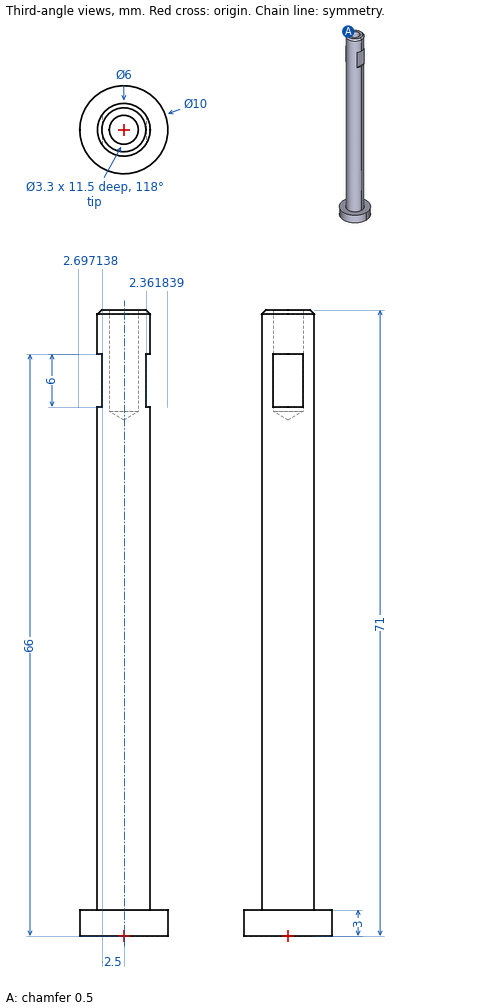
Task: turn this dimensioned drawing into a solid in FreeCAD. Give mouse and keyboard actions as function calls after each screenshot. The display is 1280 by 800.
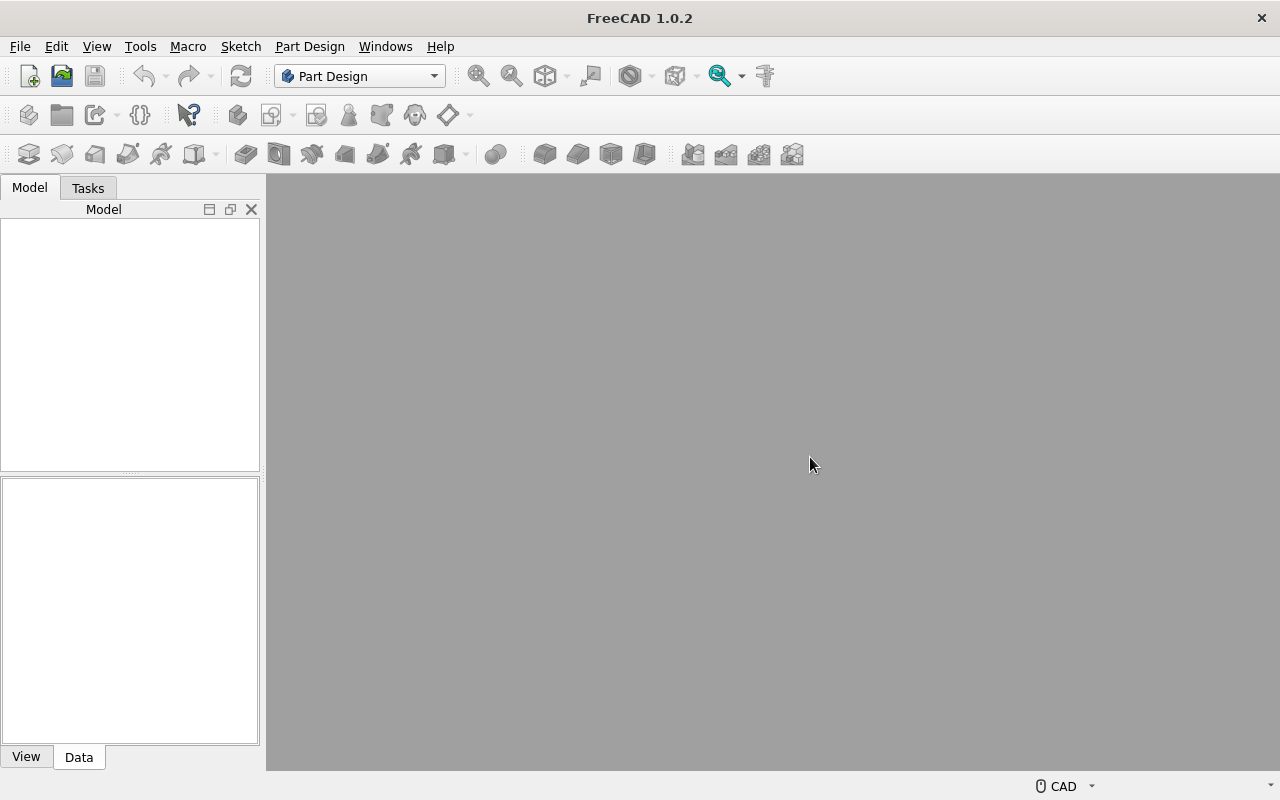
key(ctrl+n)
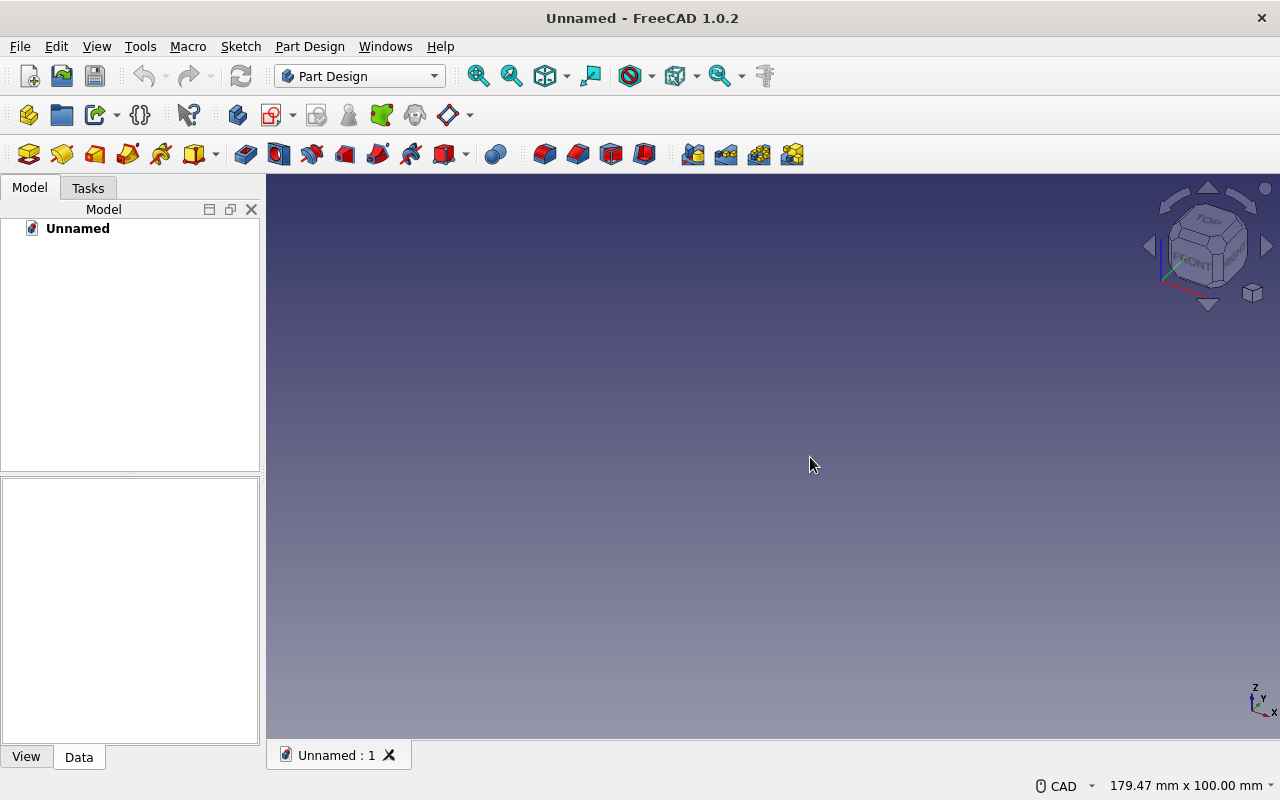
click(270, 116)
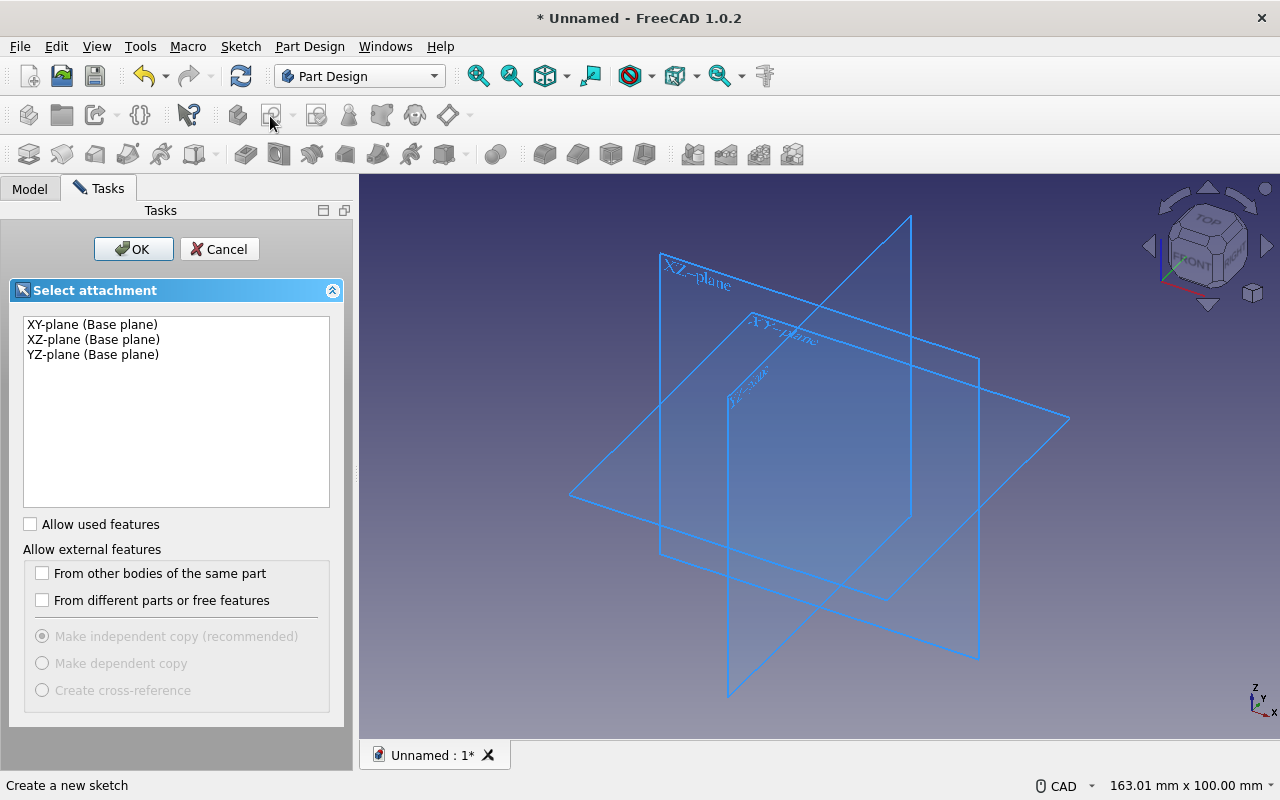
click(84, 324)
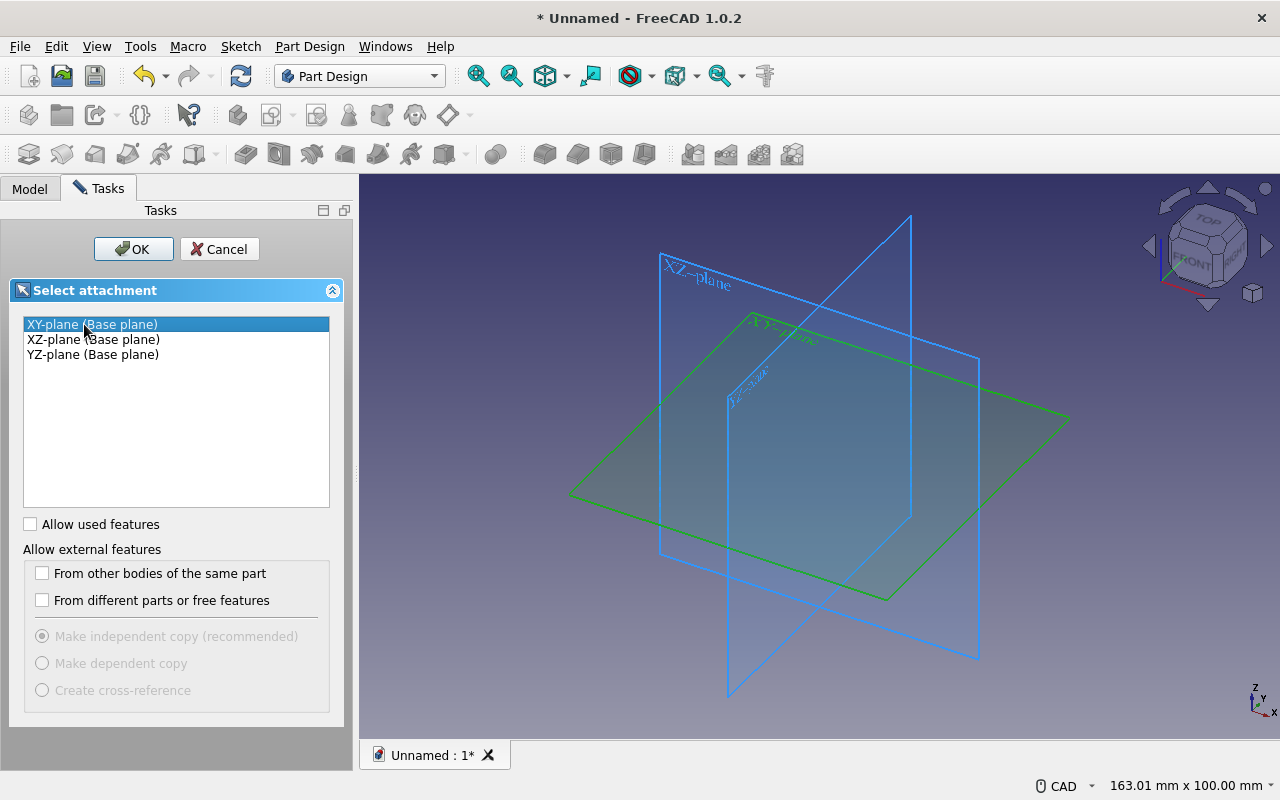
click(134, 249)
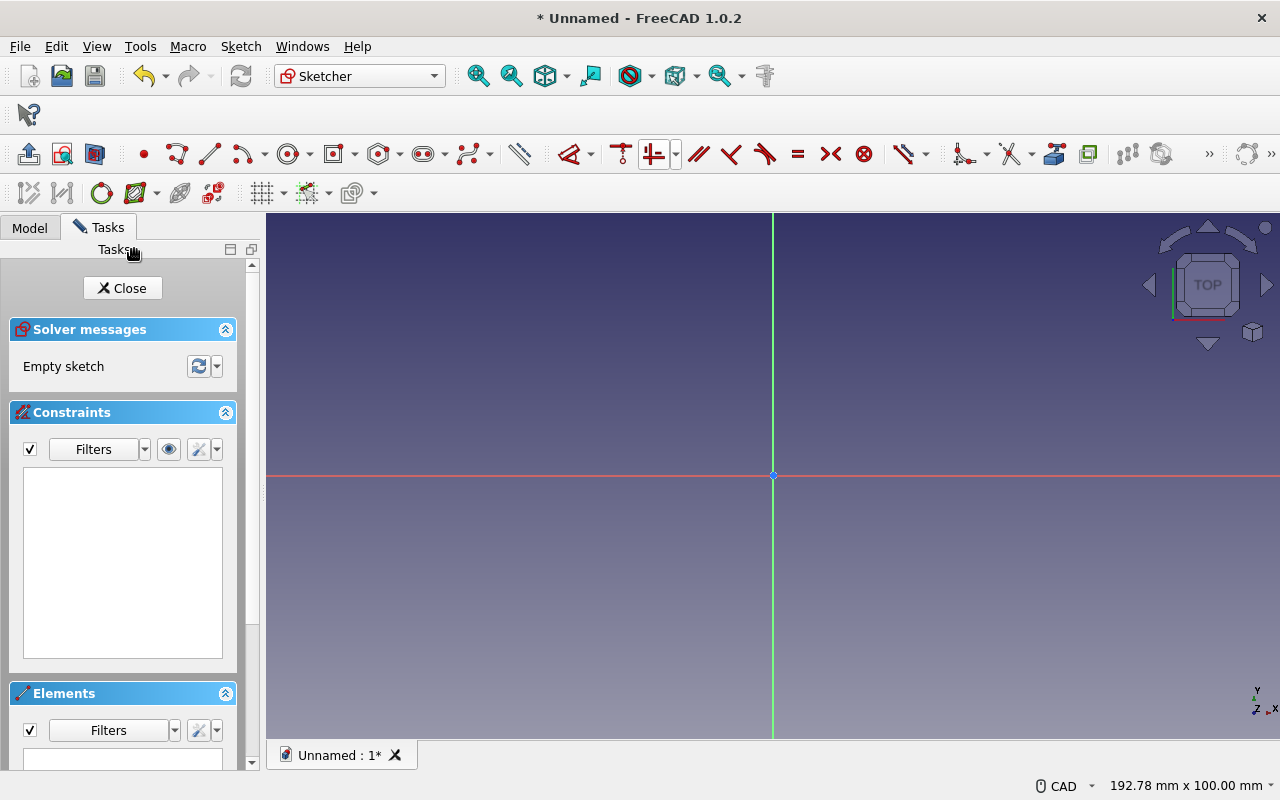
scroll(780, 476, up, 12)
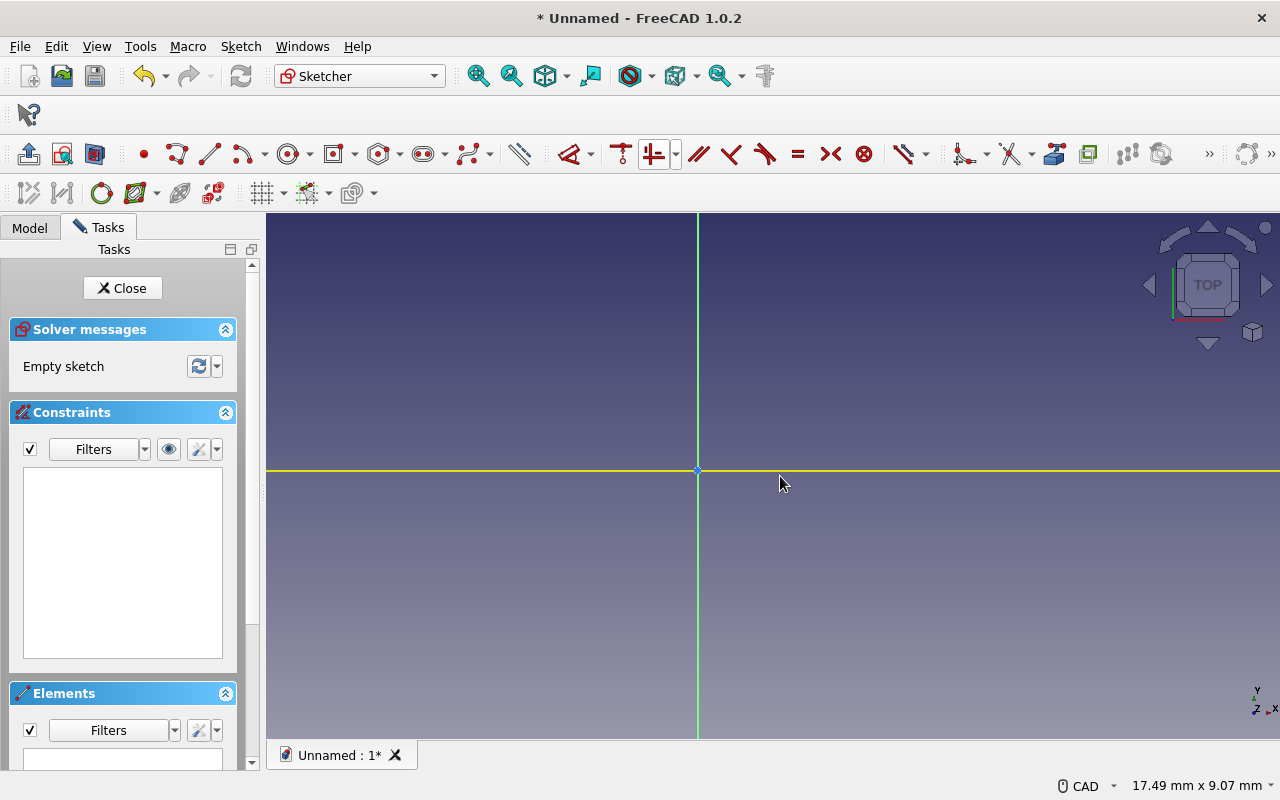
click(288, 154)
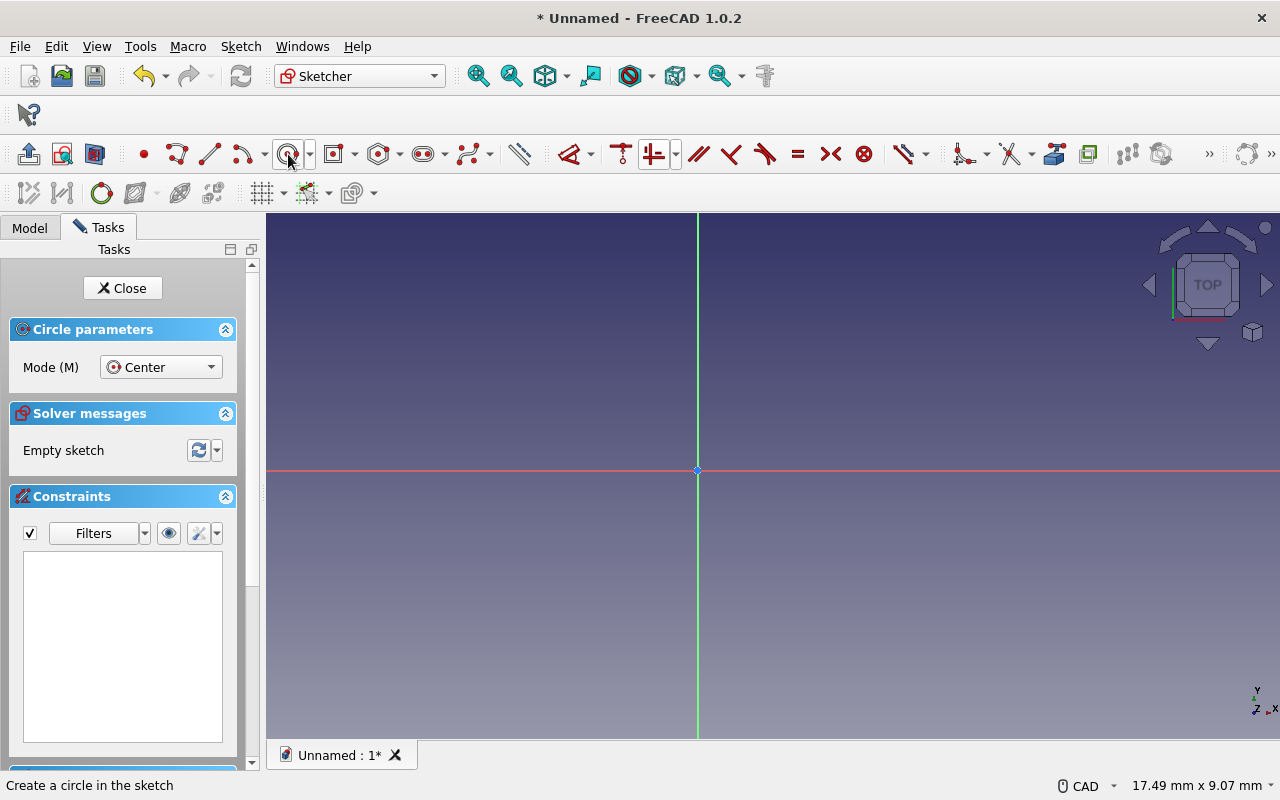
click(698, 471)
move(821, 348)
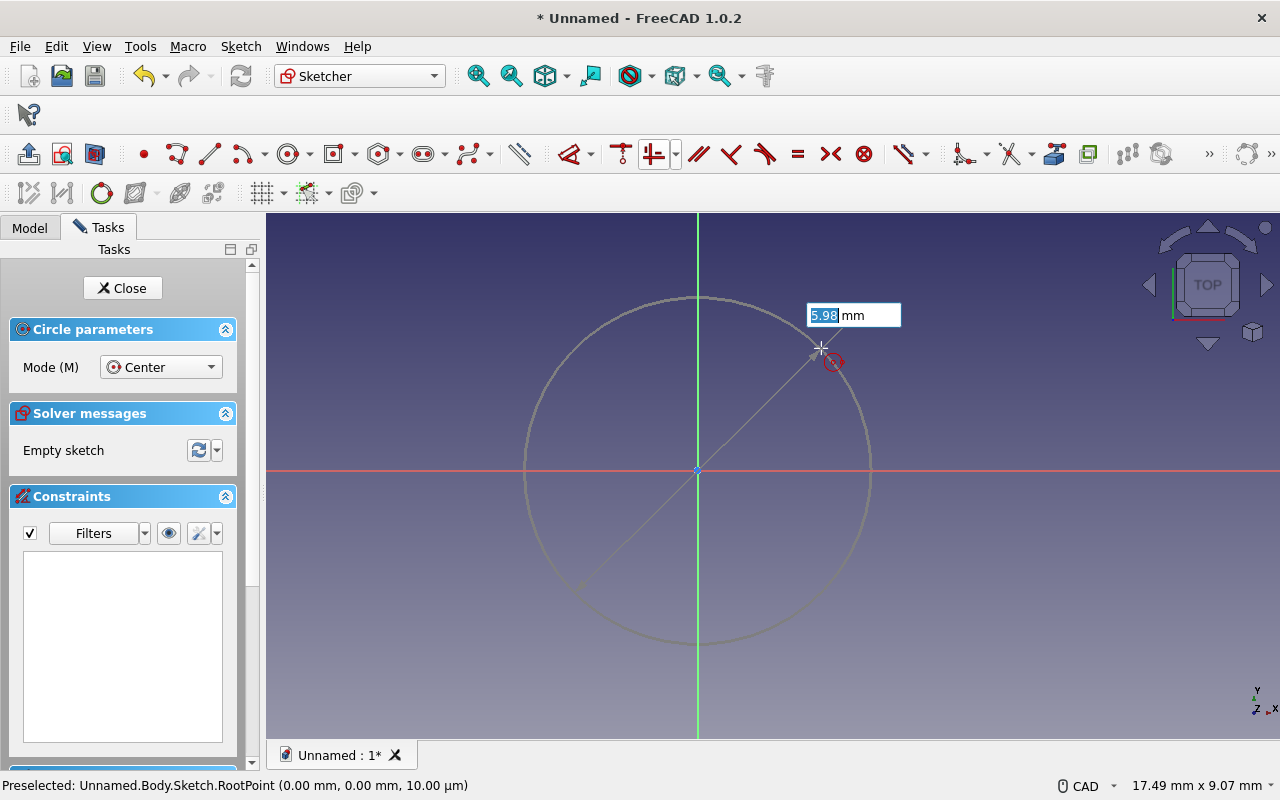
text(6)
key(Return)
key(Escape)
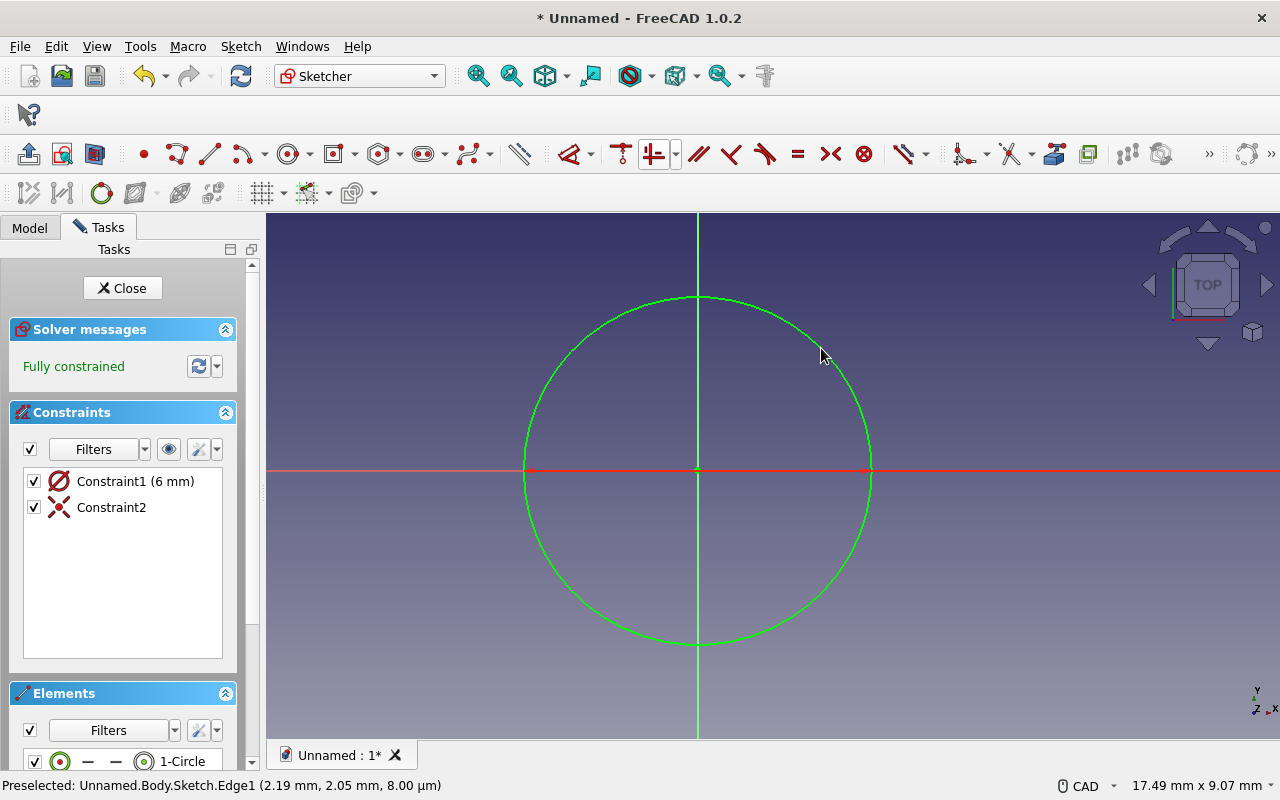
click(123, 288)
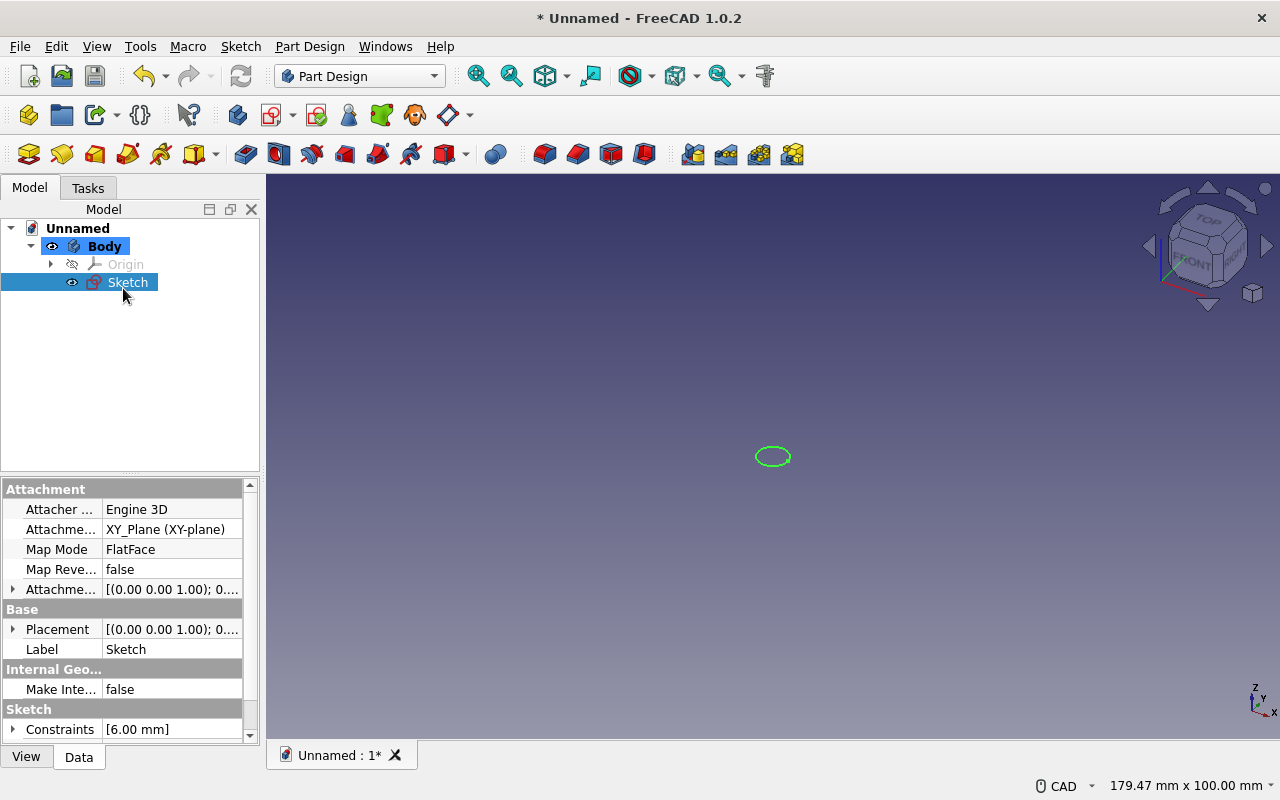
click(29, 154)